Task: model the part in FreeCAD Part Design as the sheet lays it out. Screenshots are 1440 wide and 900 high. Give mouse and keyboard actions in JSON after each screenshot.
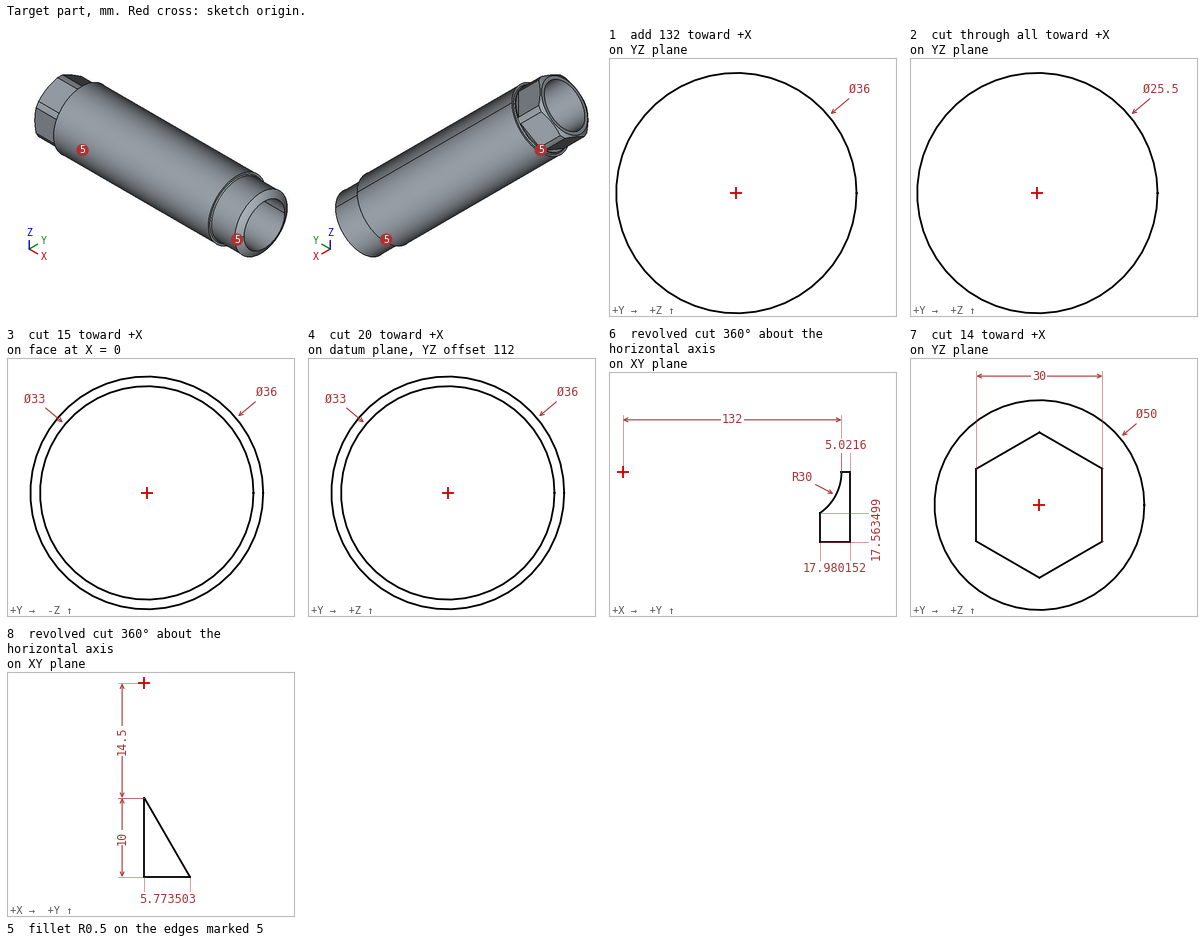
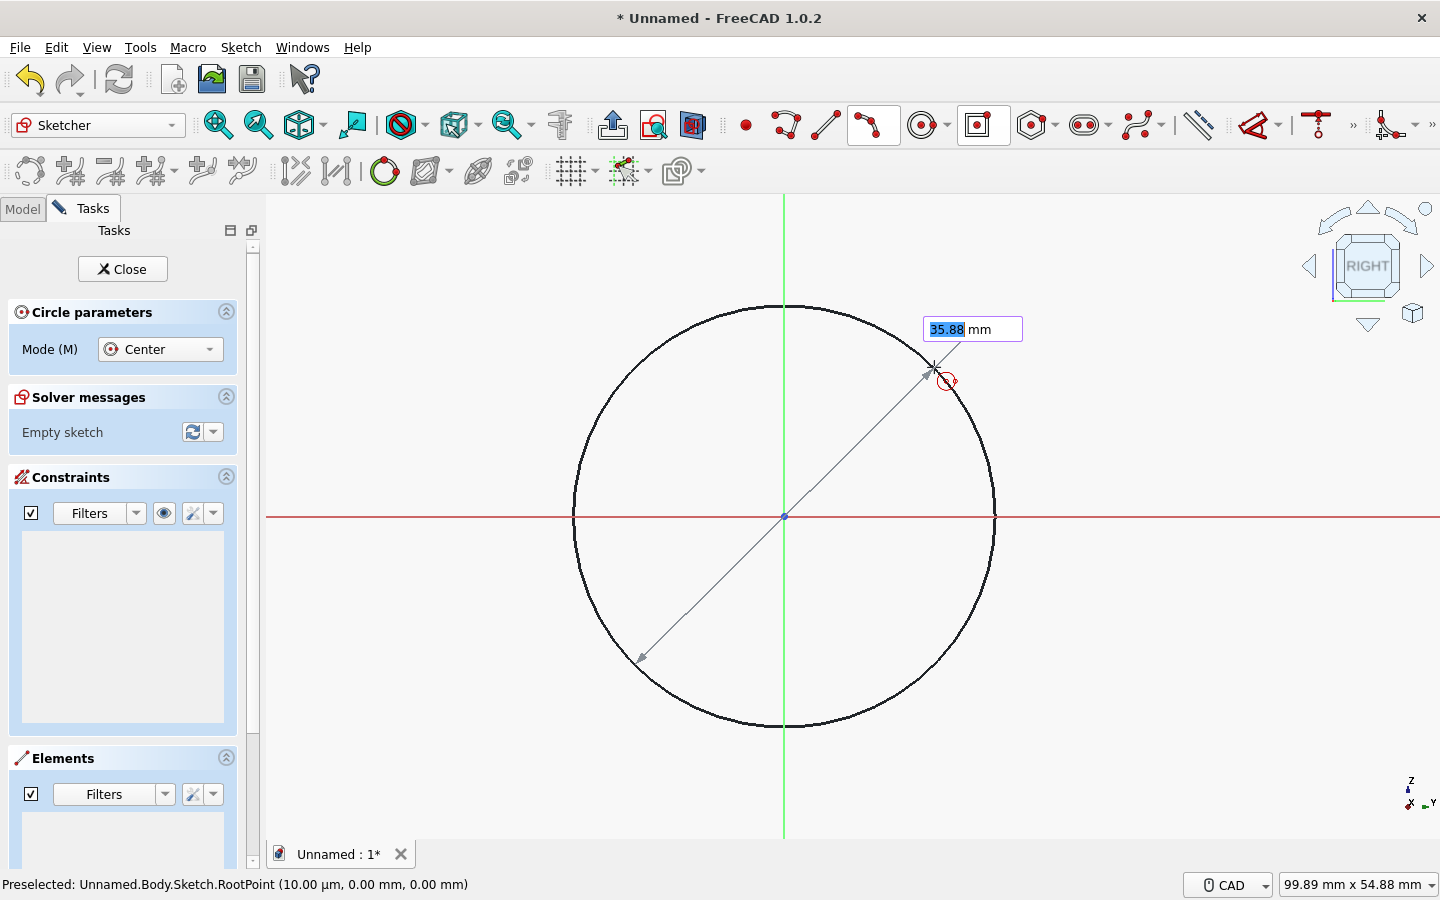
{"action": "type", "text": "36"}
{"action": "key", "text": "Return"}
{"action": "key", "text": "Escape"}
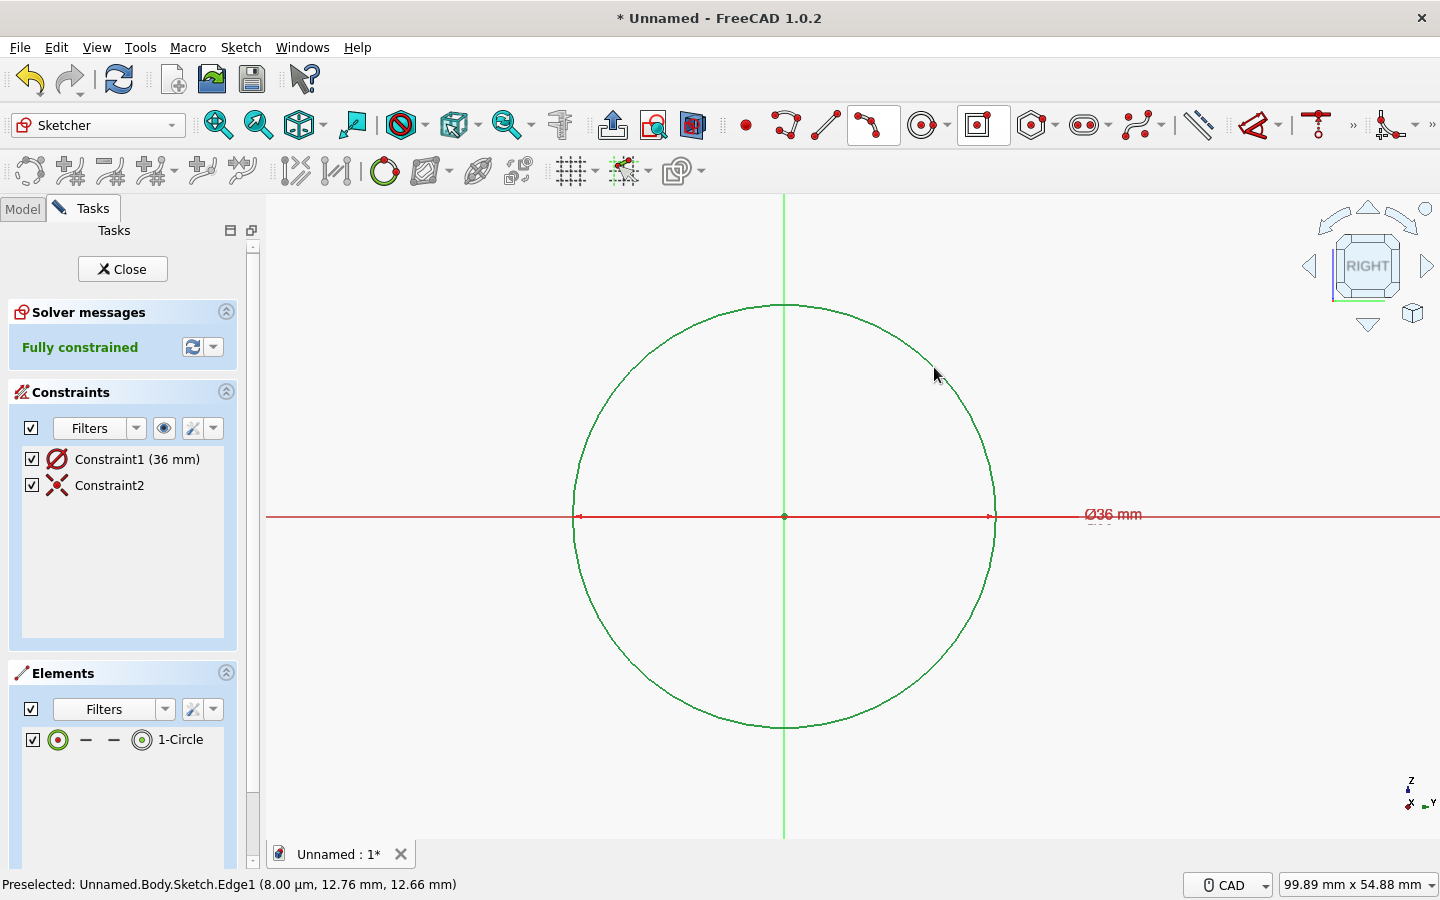
{"action": "left_click", "coordinate": [123, 269]}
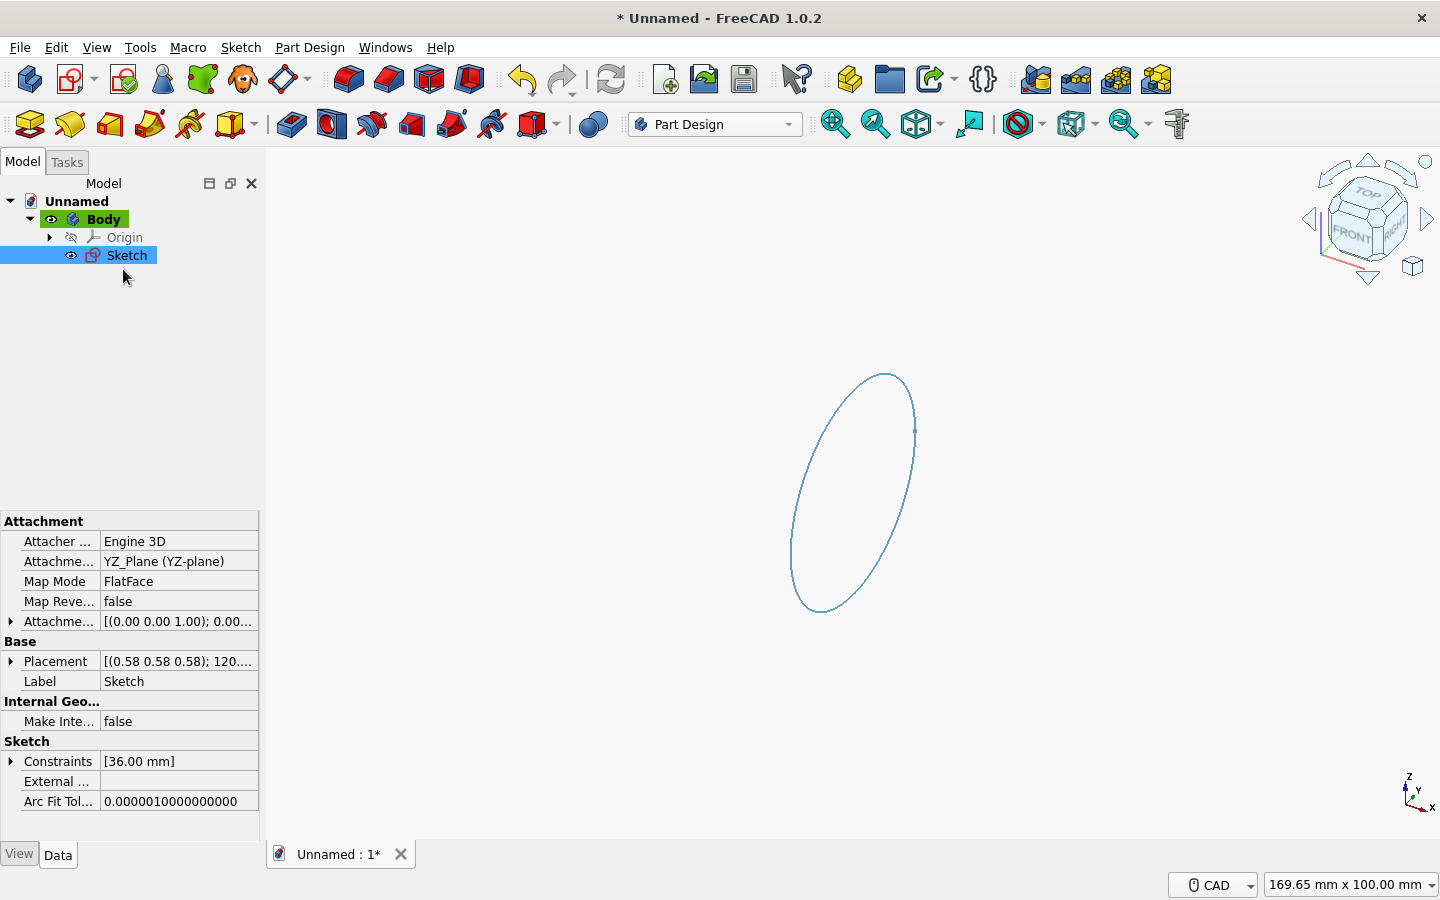
{"action": "left_click", "coordinate": [30, 124]}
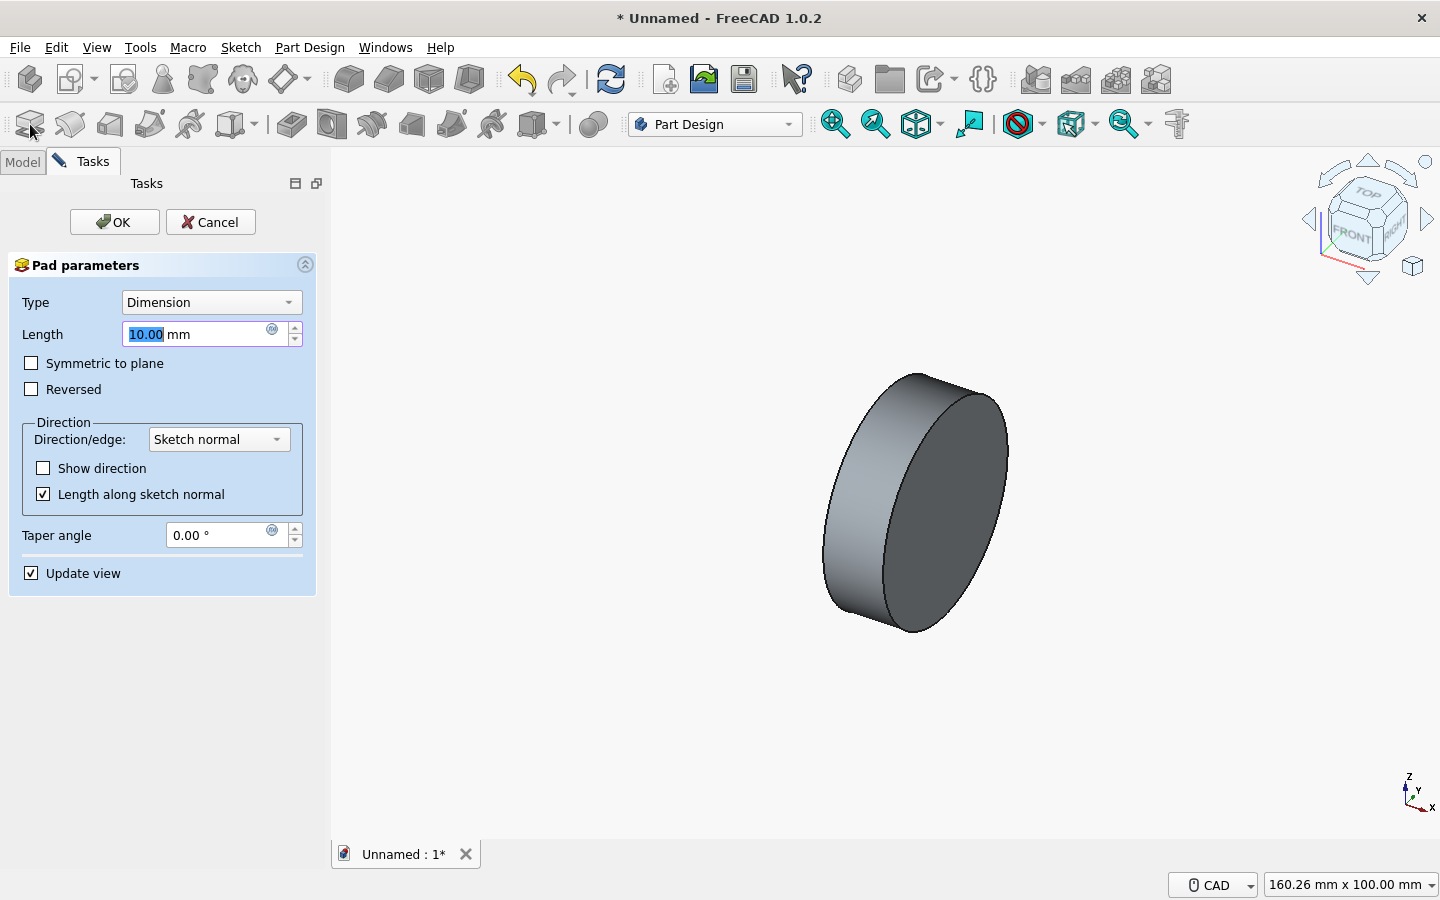
{"action": "type", "text": "132"}
{"action": "key", "text": "Tab"}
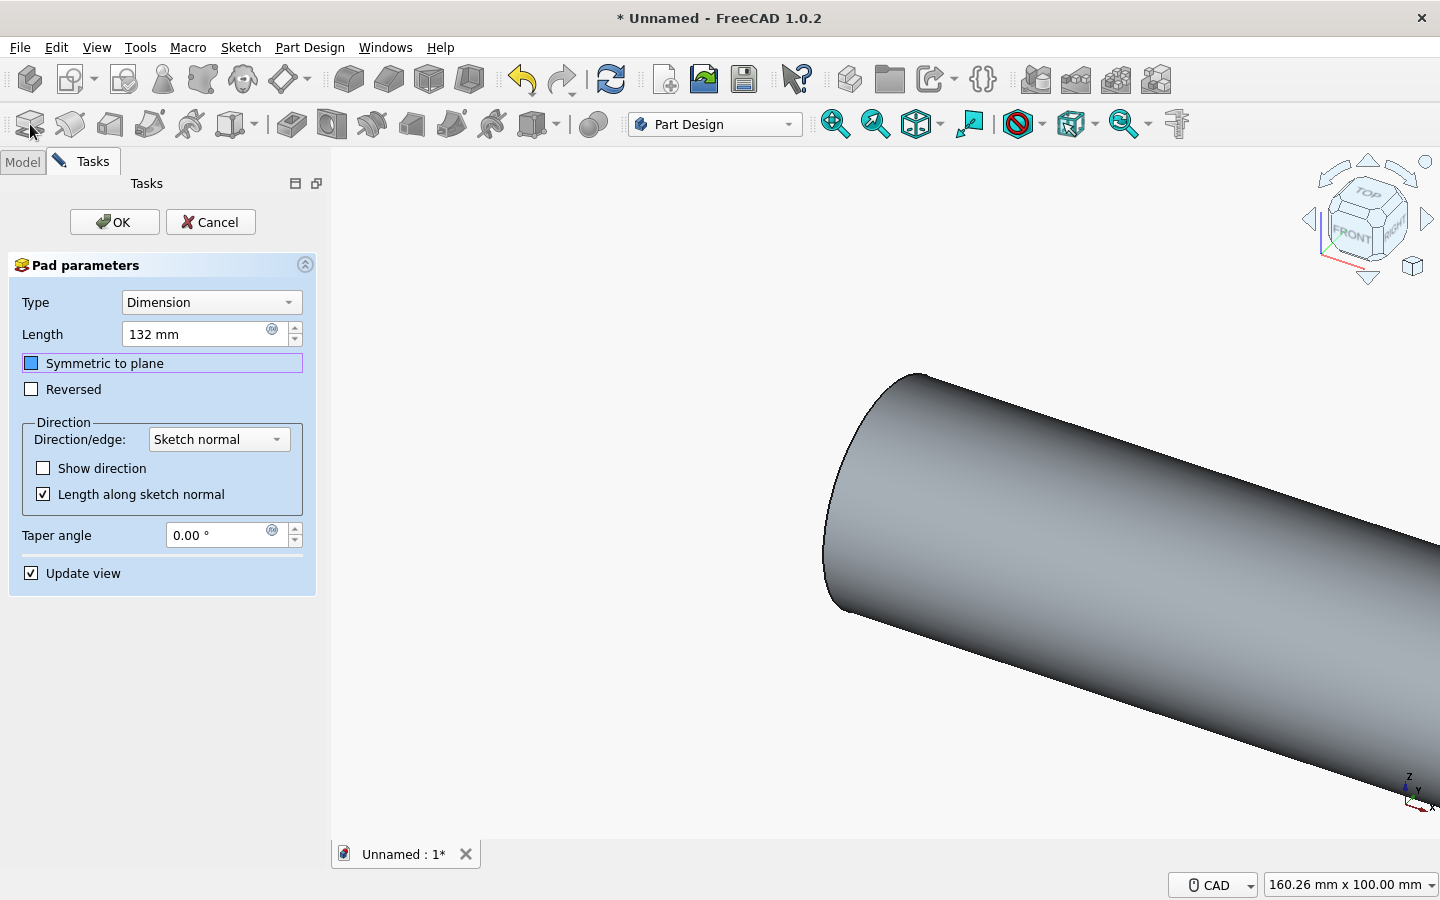
{"action": "left_click", "coordinate": [115, 222]}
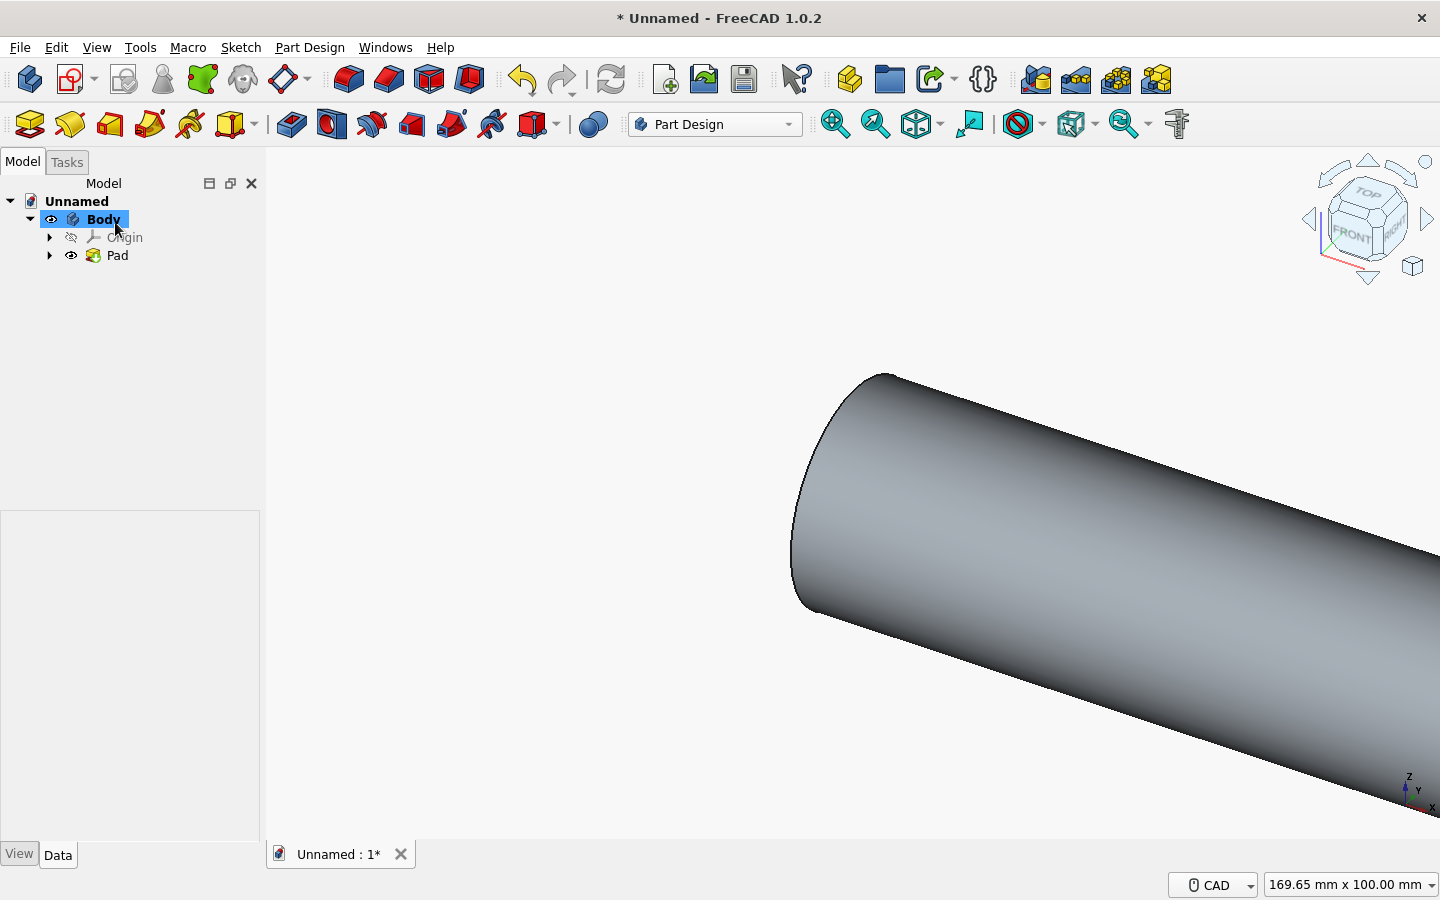
{"action": "left_click", "coordinate": [836, 124]}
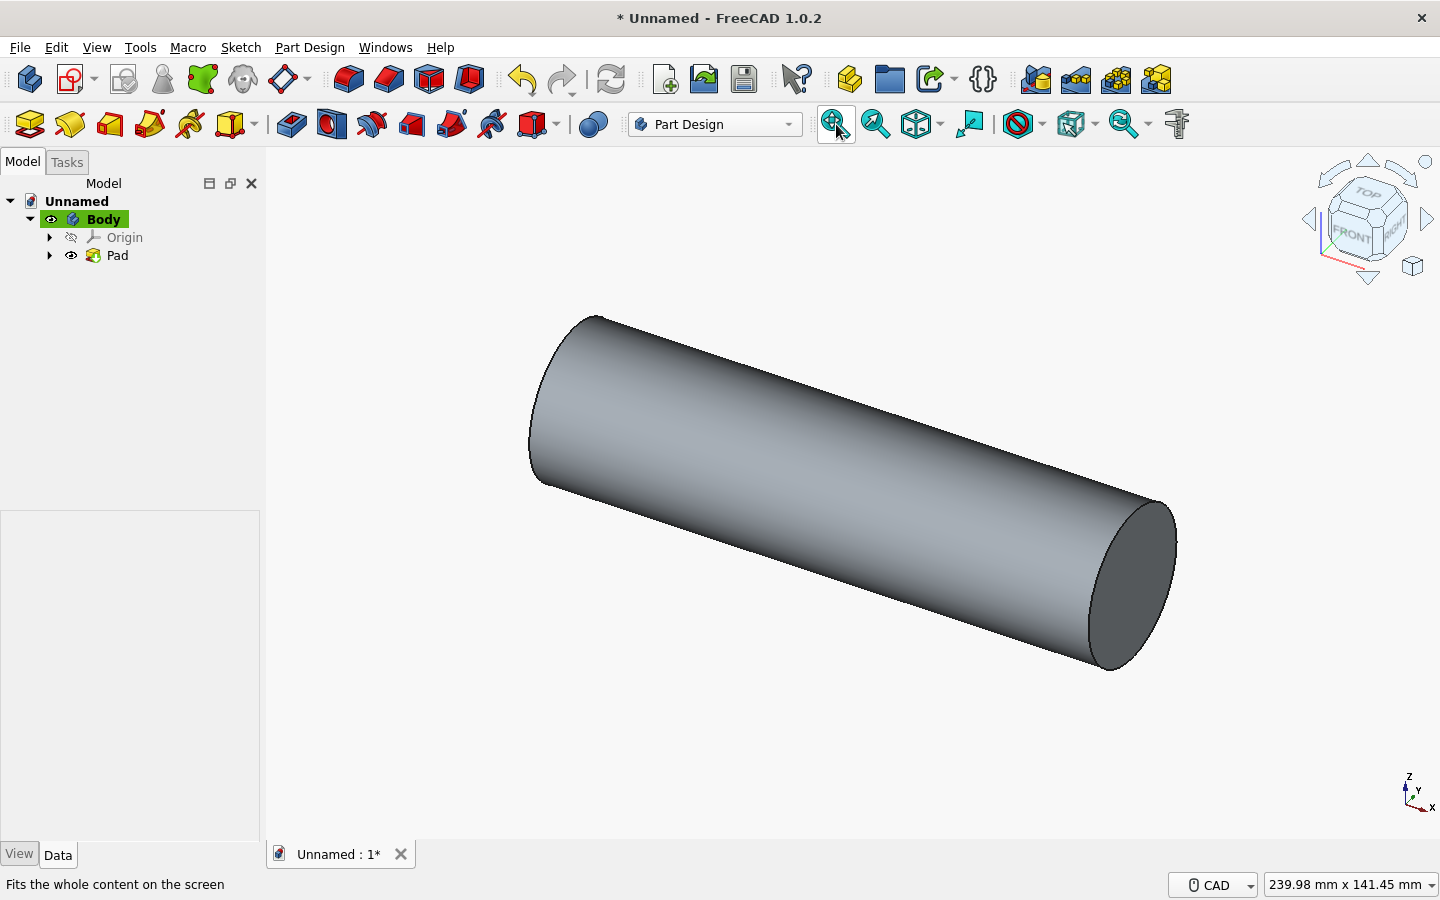
{"action": "left_click", "coordinate": [70, 80]}